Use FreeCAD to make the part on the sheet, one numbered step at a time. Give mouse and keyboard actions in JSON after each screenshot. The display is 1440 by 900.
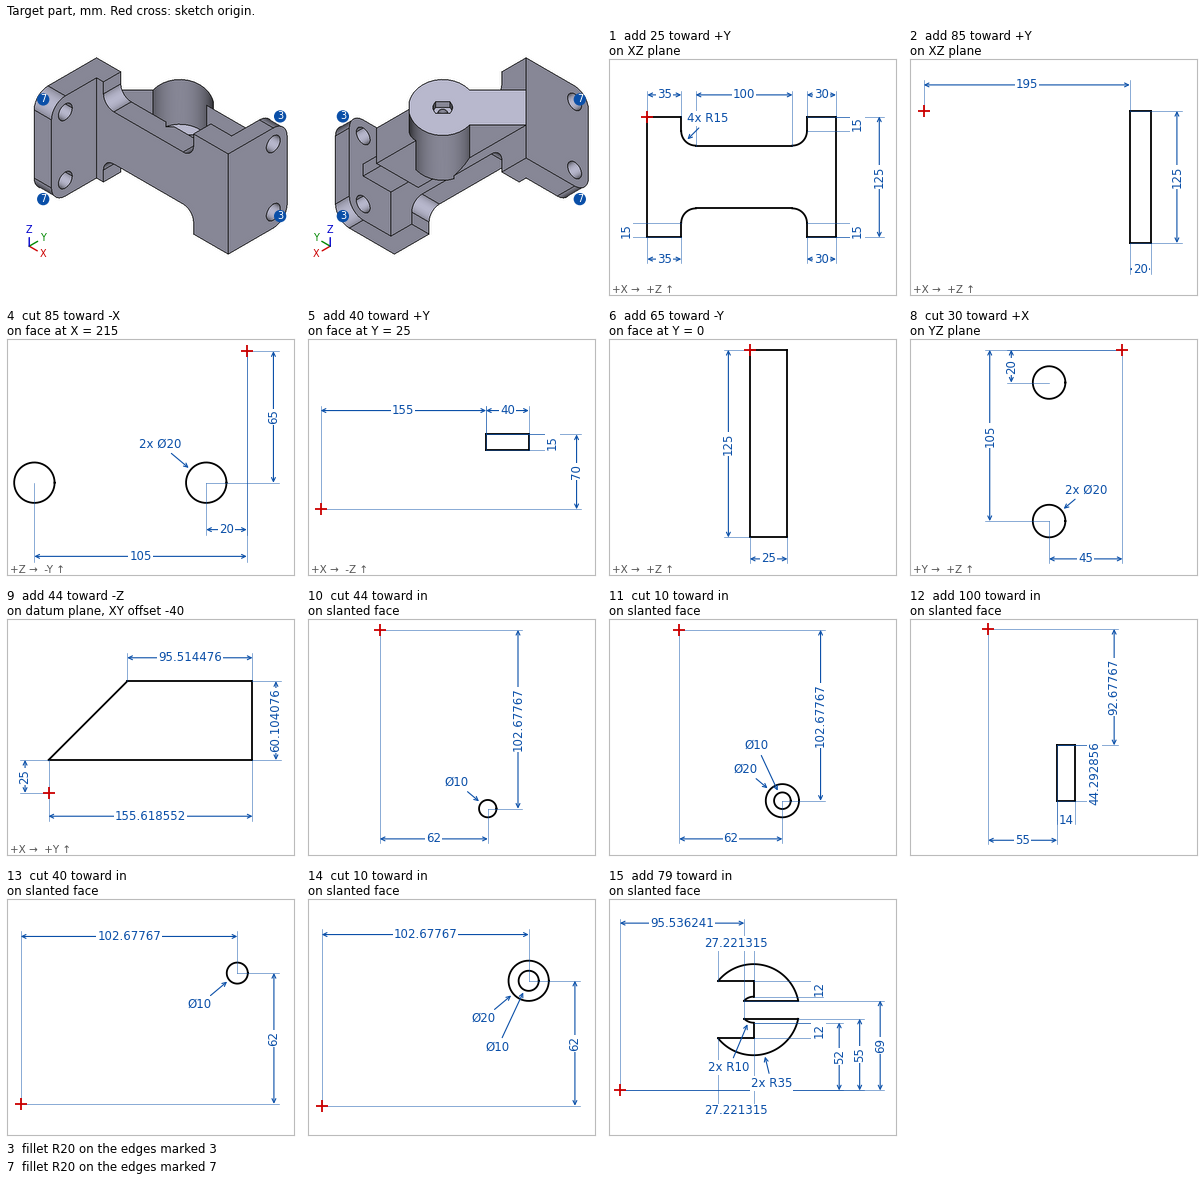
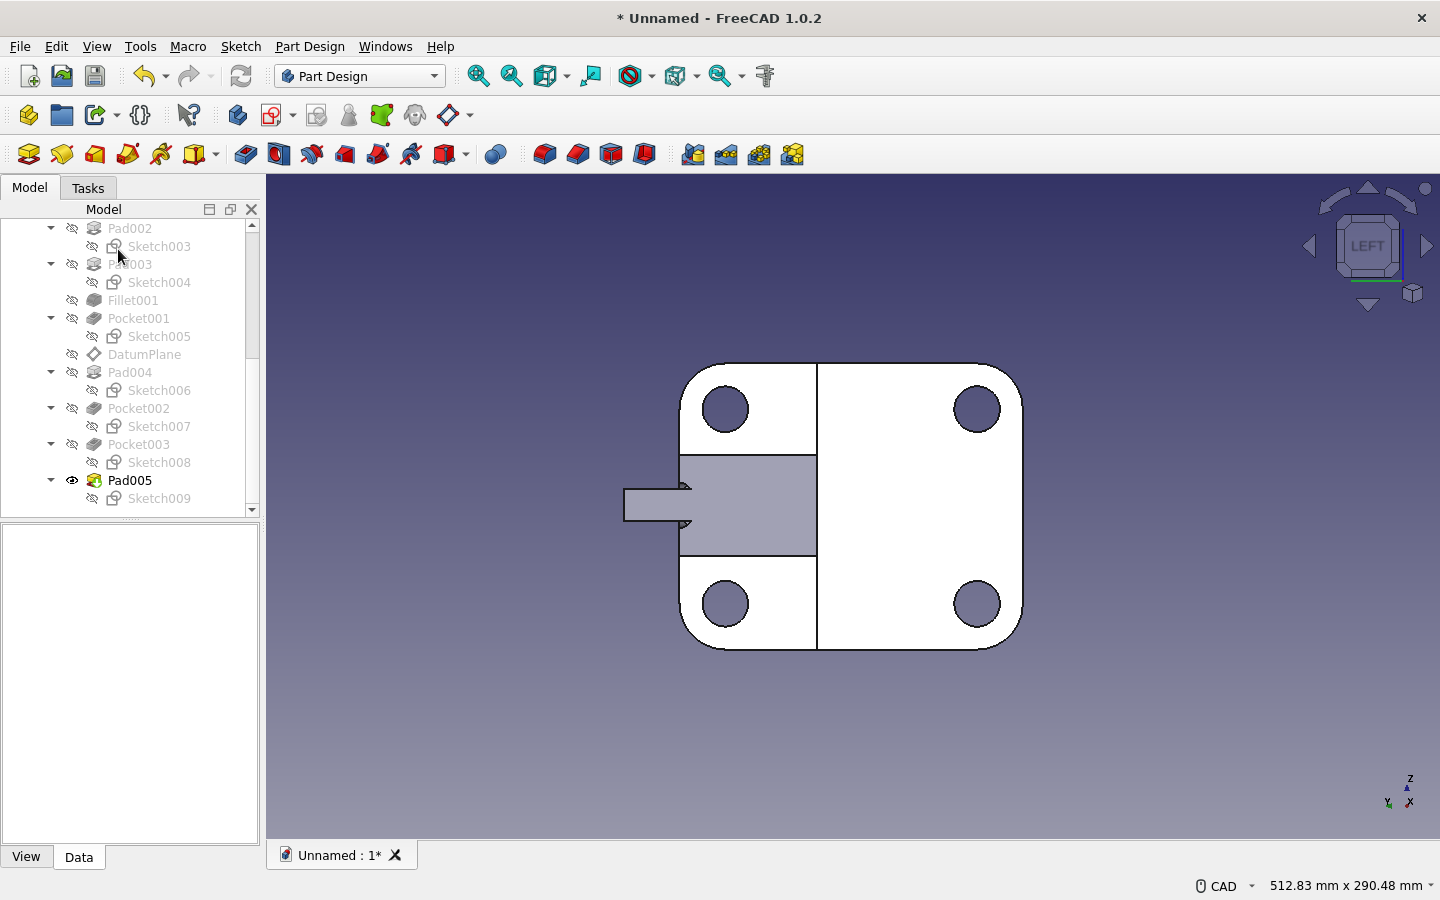
{"action": "left_click", "coordinate": [479, 76]}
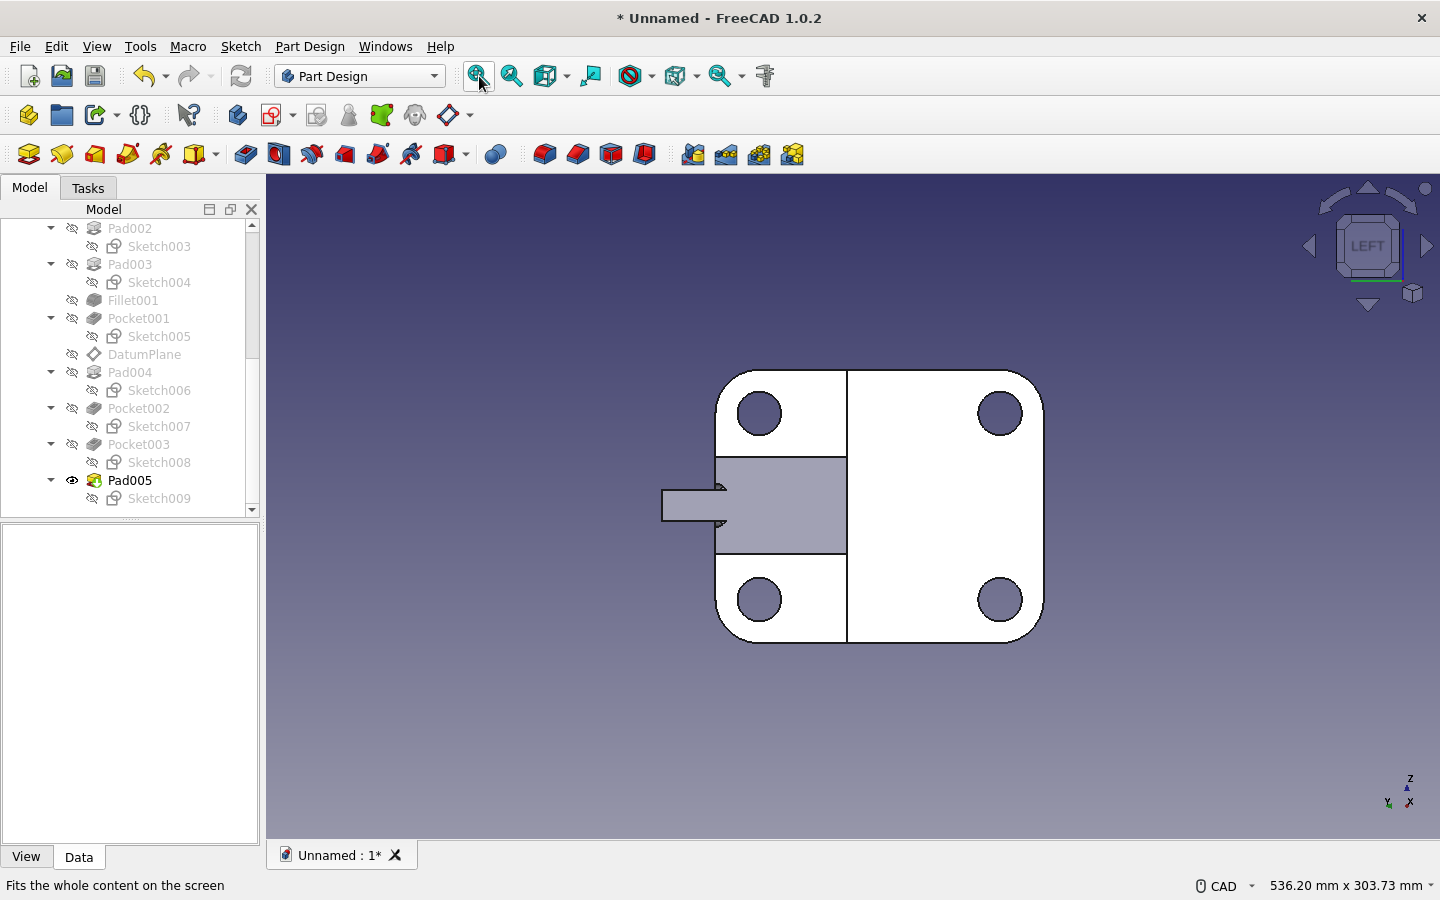
{"action": "left_click", "coordinate": [781, 504]}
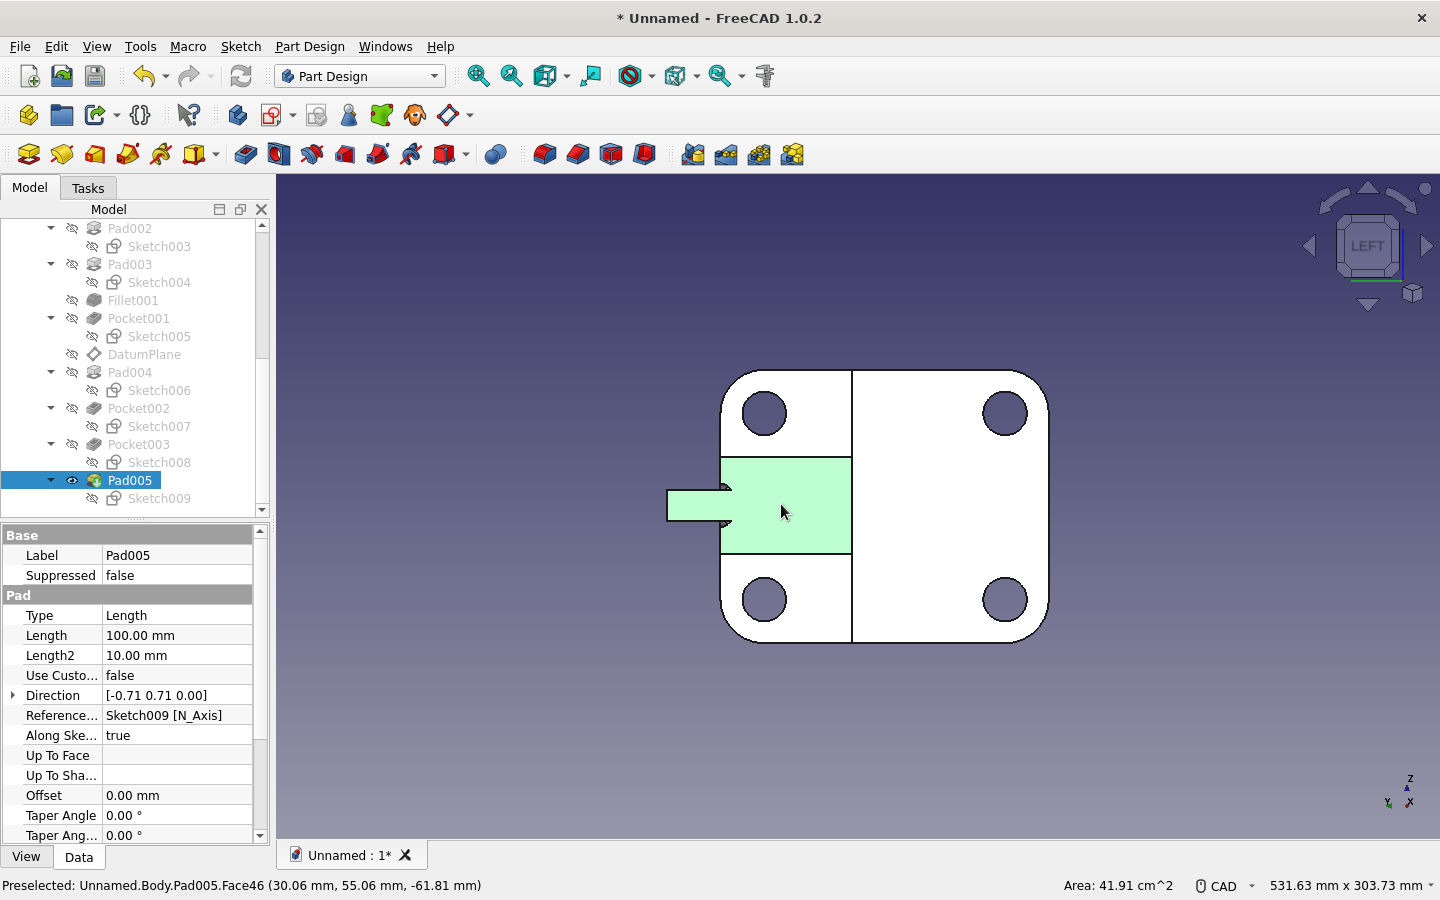
{"action": "left_click", "coordinate": [270, 116]}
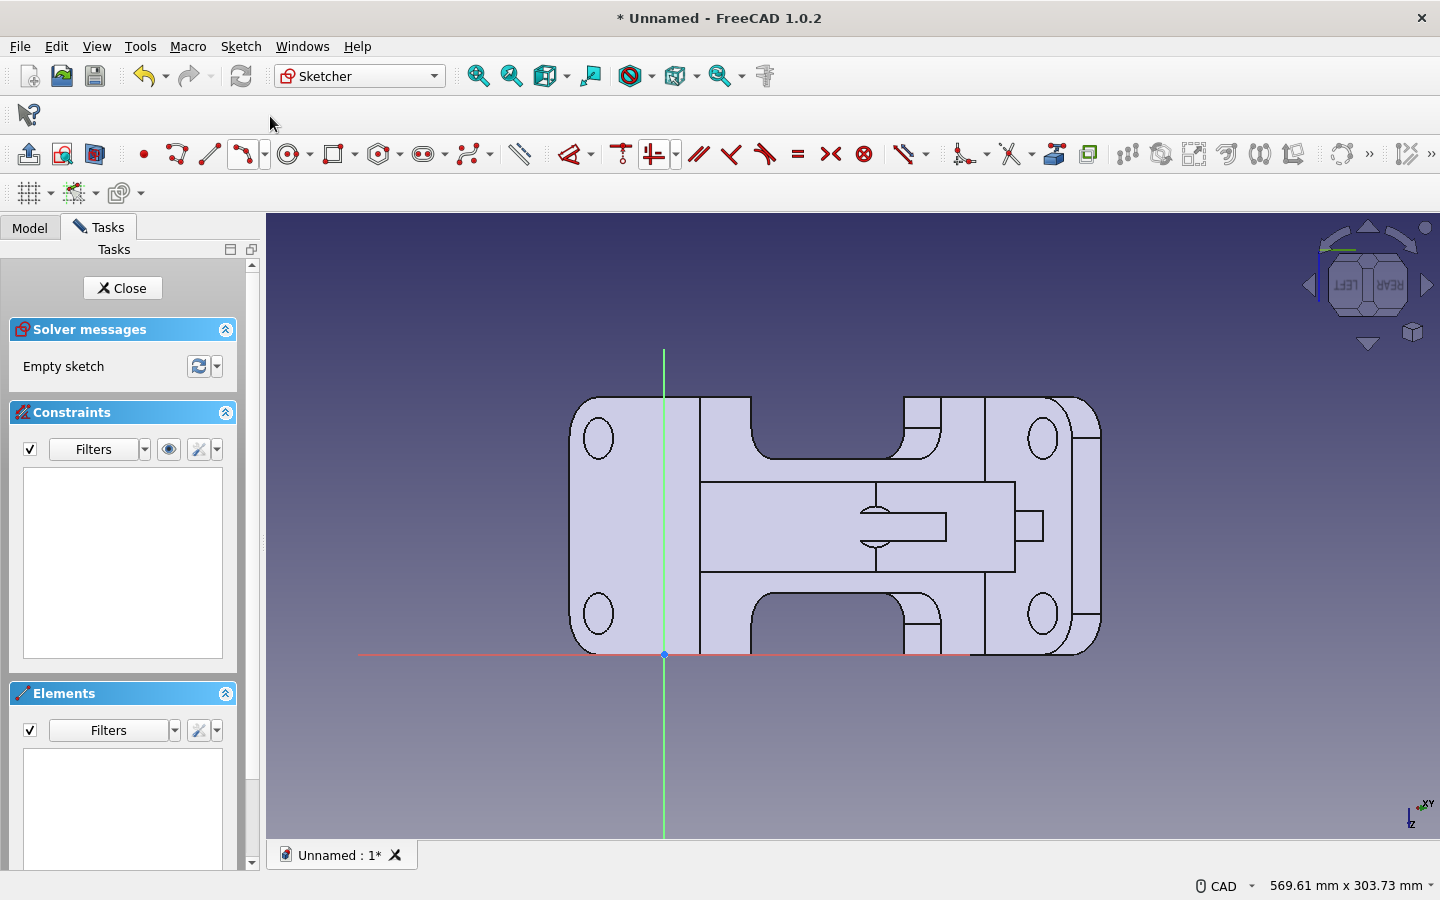
{"action": "left_click", "coordinate": [95, 154]}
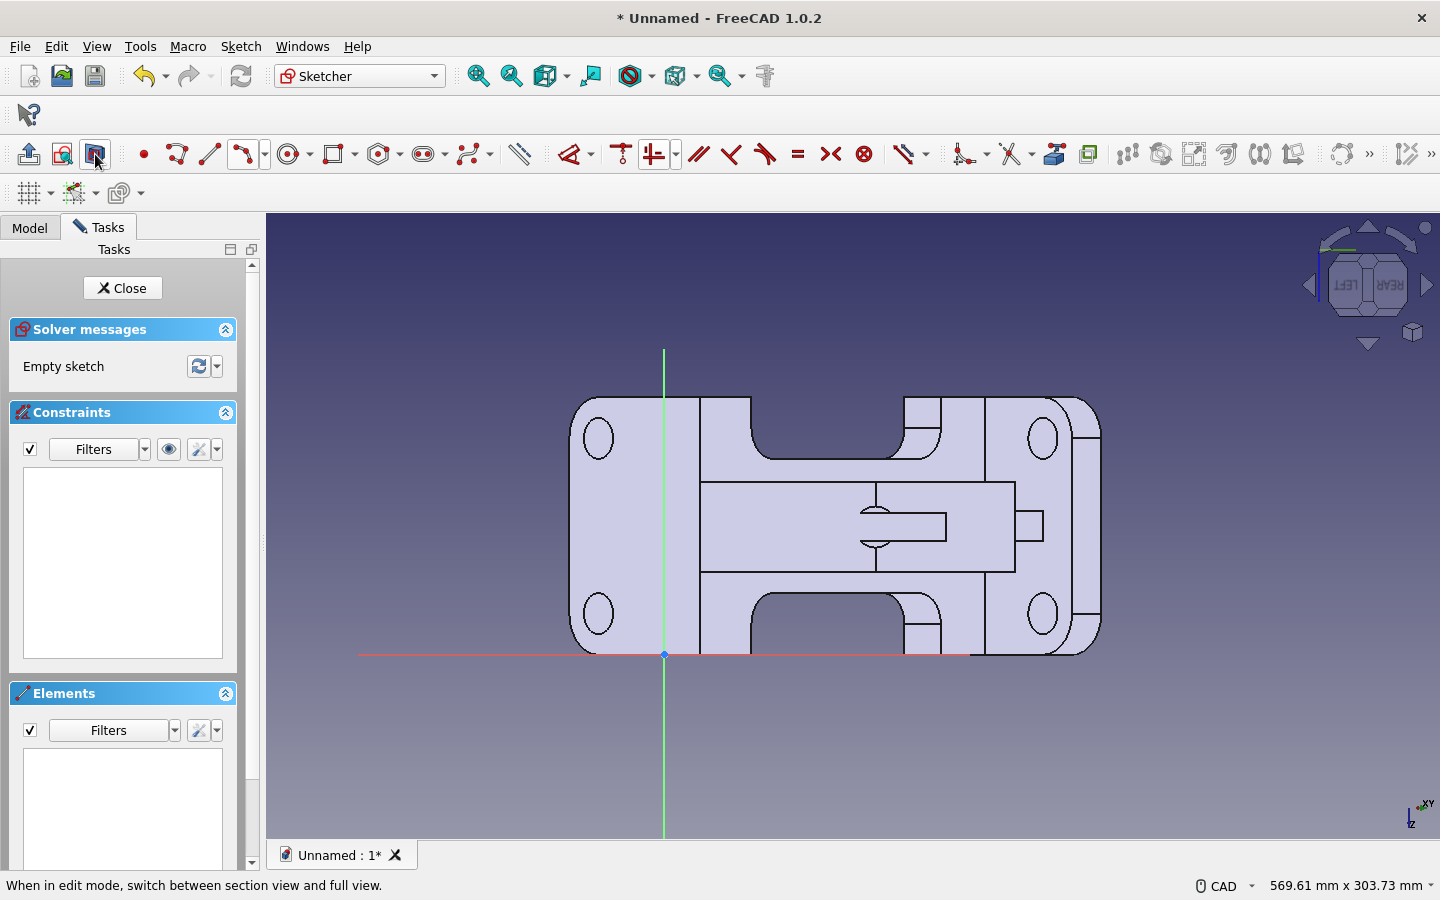
{"action": "scroll", "coordinate": [880, 527], "scroll_direction": "up", "scroll_amount": 15}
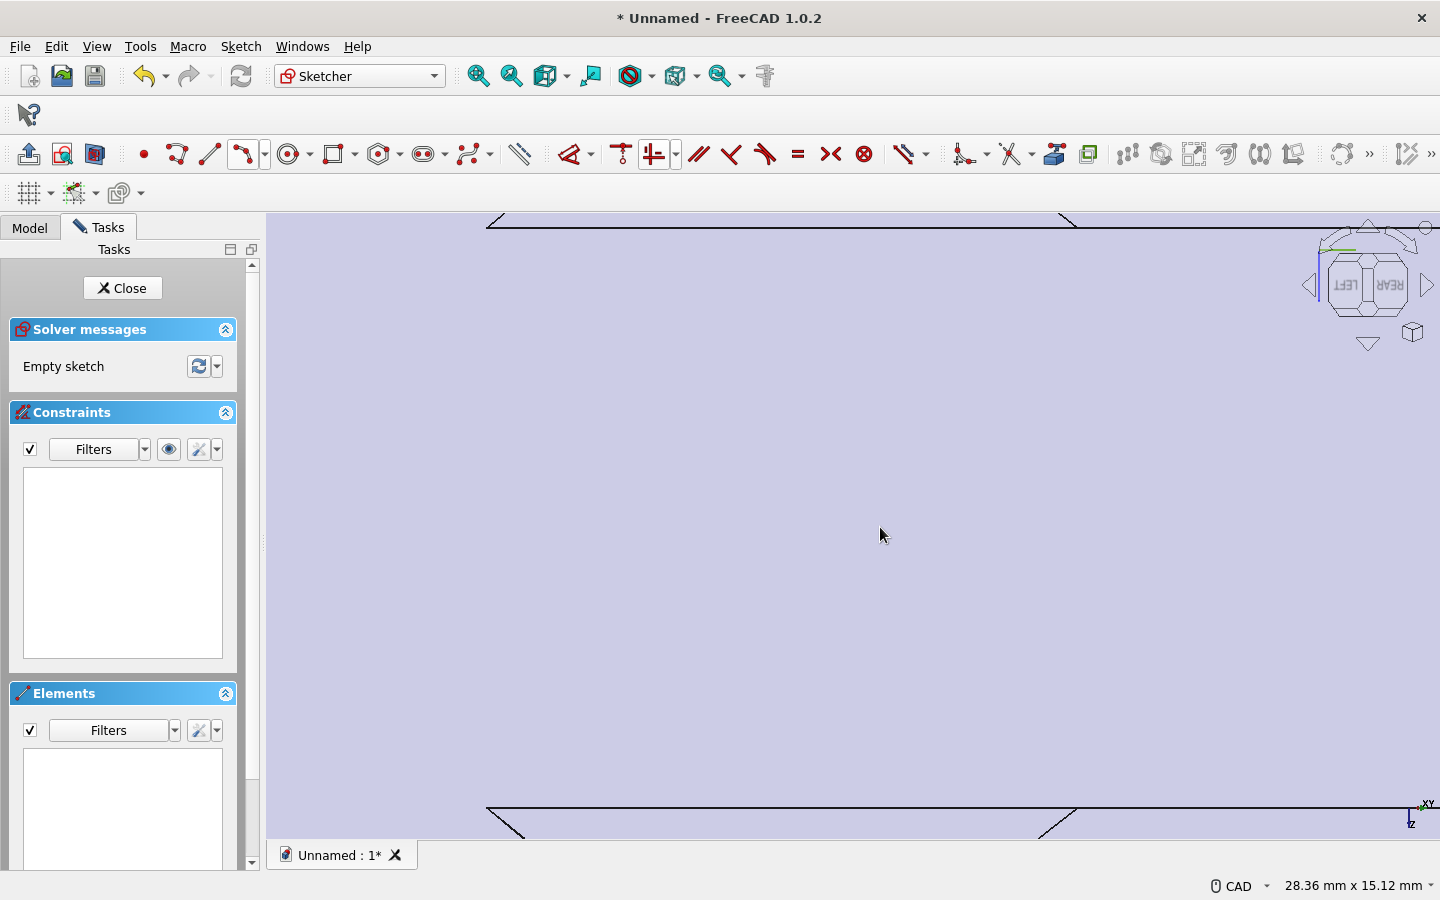
{"action": "left_click", "coordinate": [288, 154]}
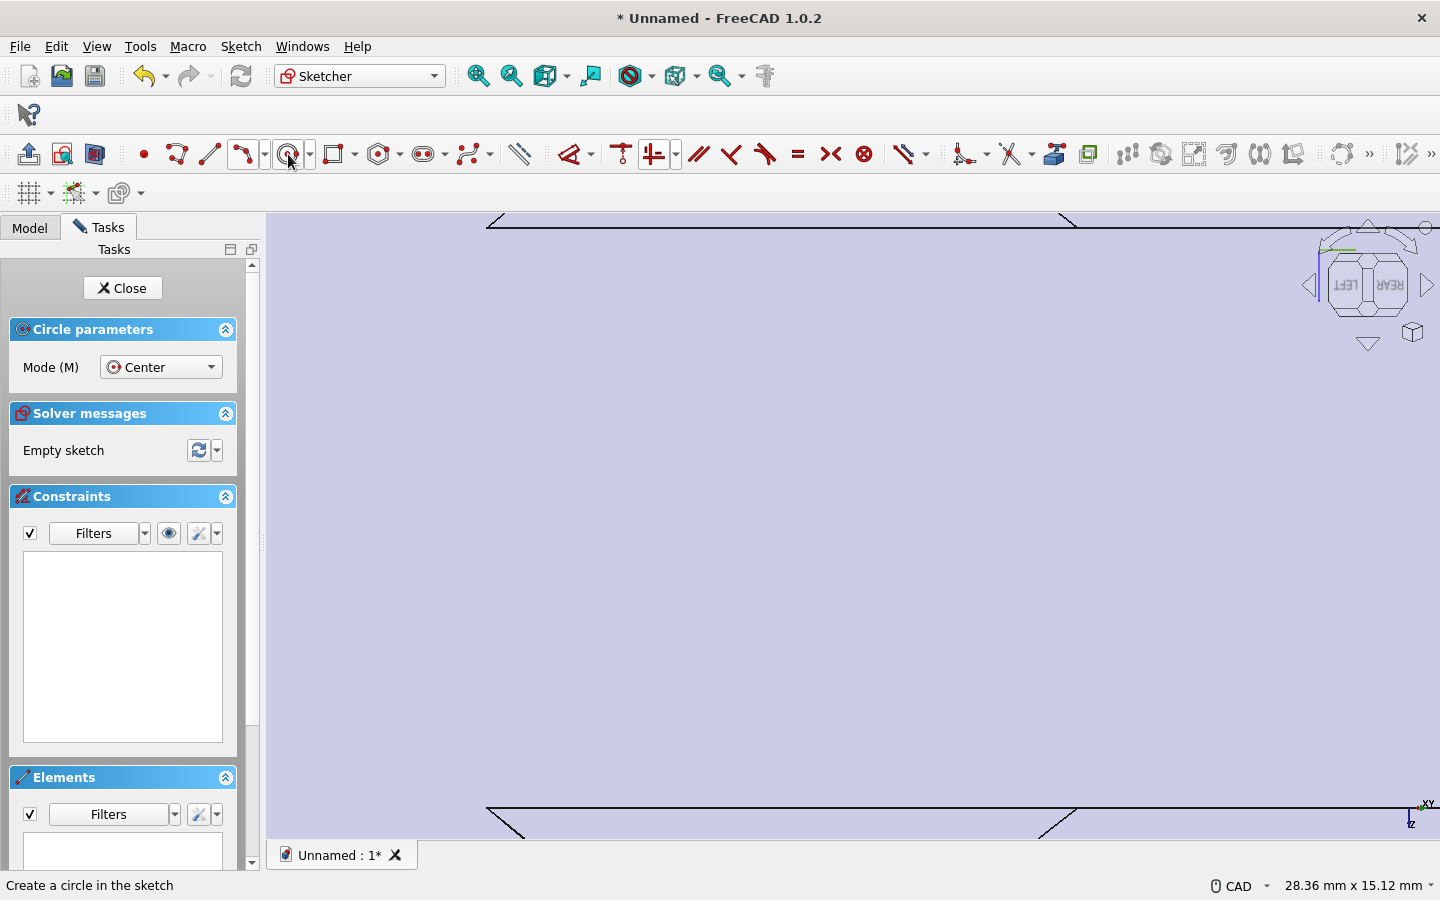
{"action": "left_click", "coordinate": [782, 518]}
{"action": "left_click", "coordinate": [929, 372]}
{"action": "key", "text": "Escape"}